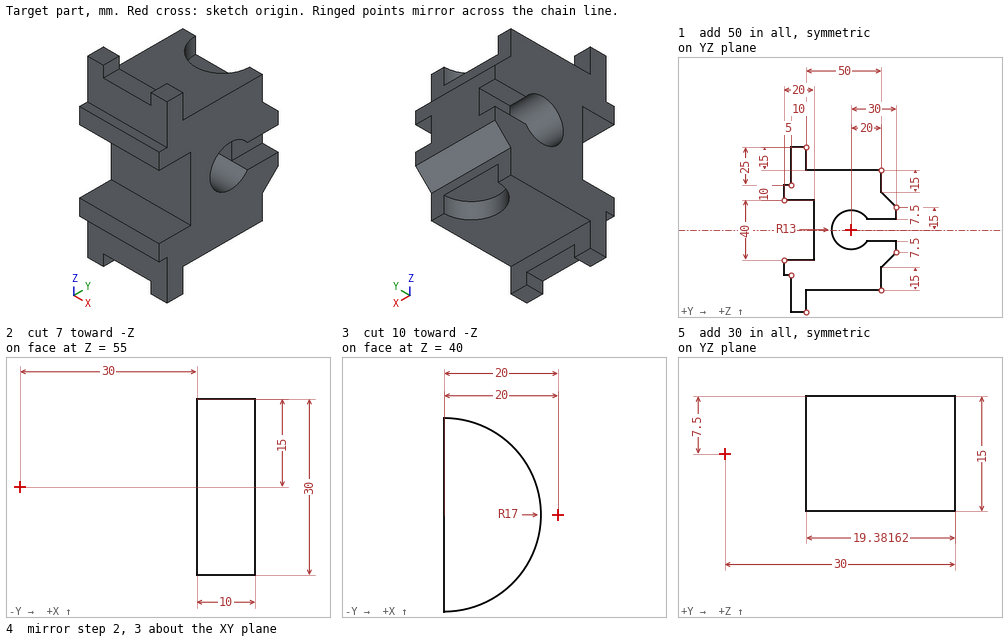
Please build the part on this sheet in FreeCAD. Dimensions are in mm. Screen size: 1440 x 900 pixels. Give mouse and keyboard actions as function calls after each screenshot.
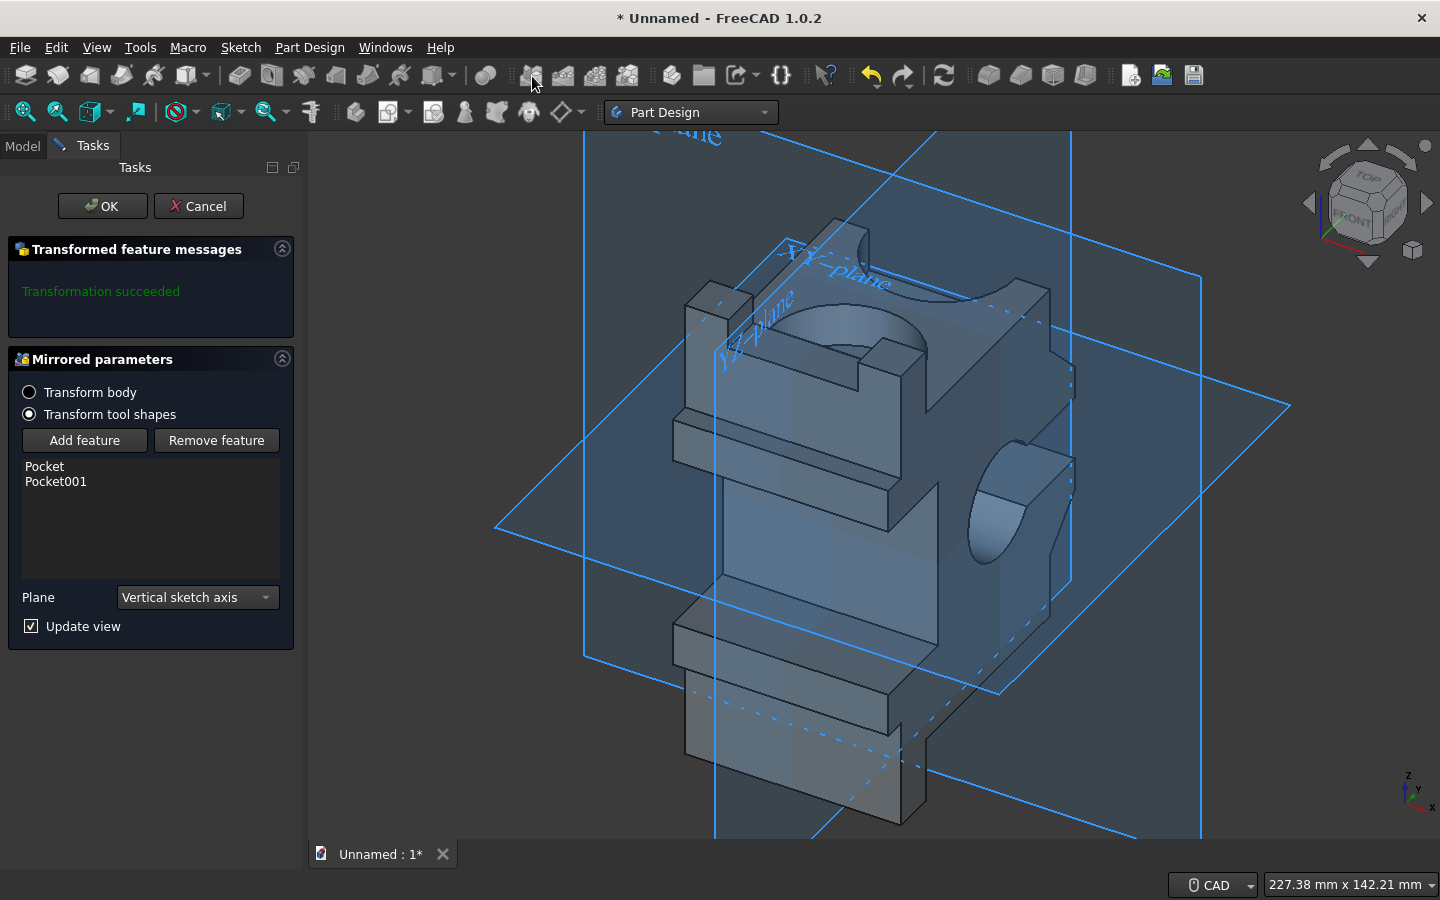
click(198, 598)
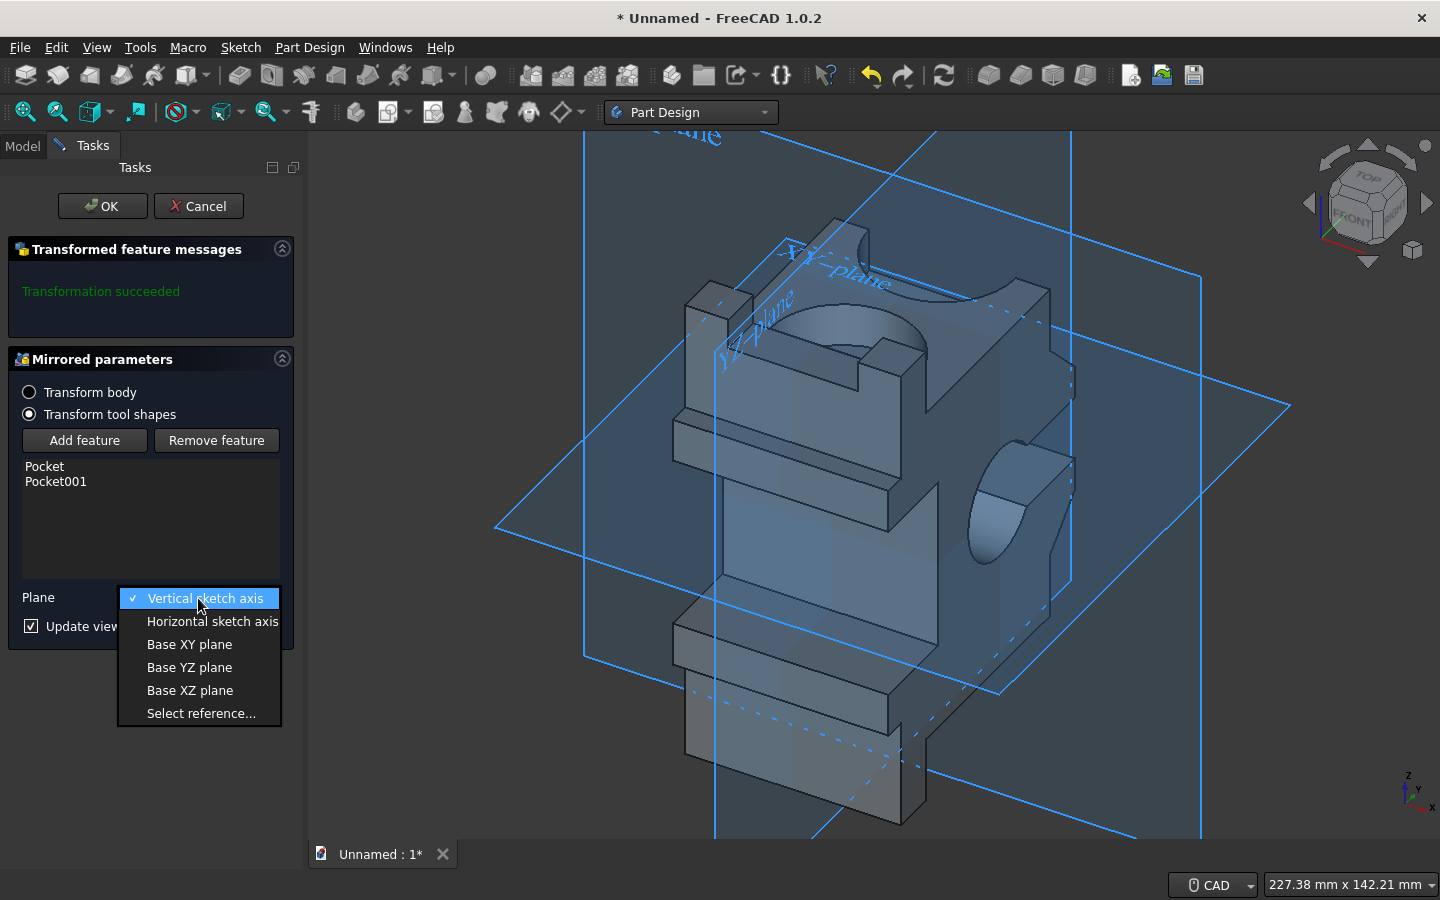
click(198, 644)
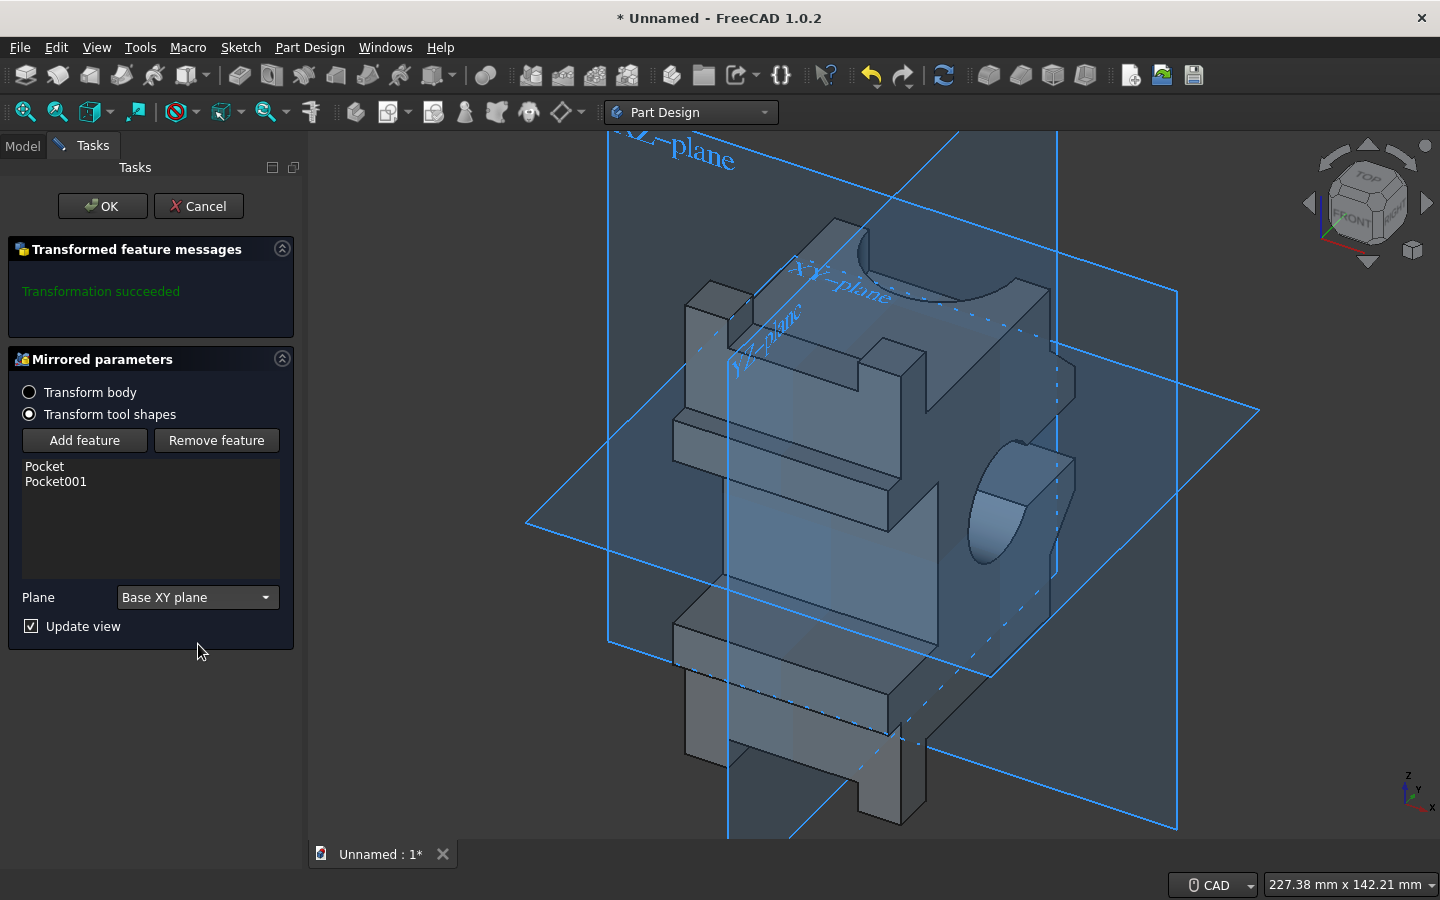
click(103, 206)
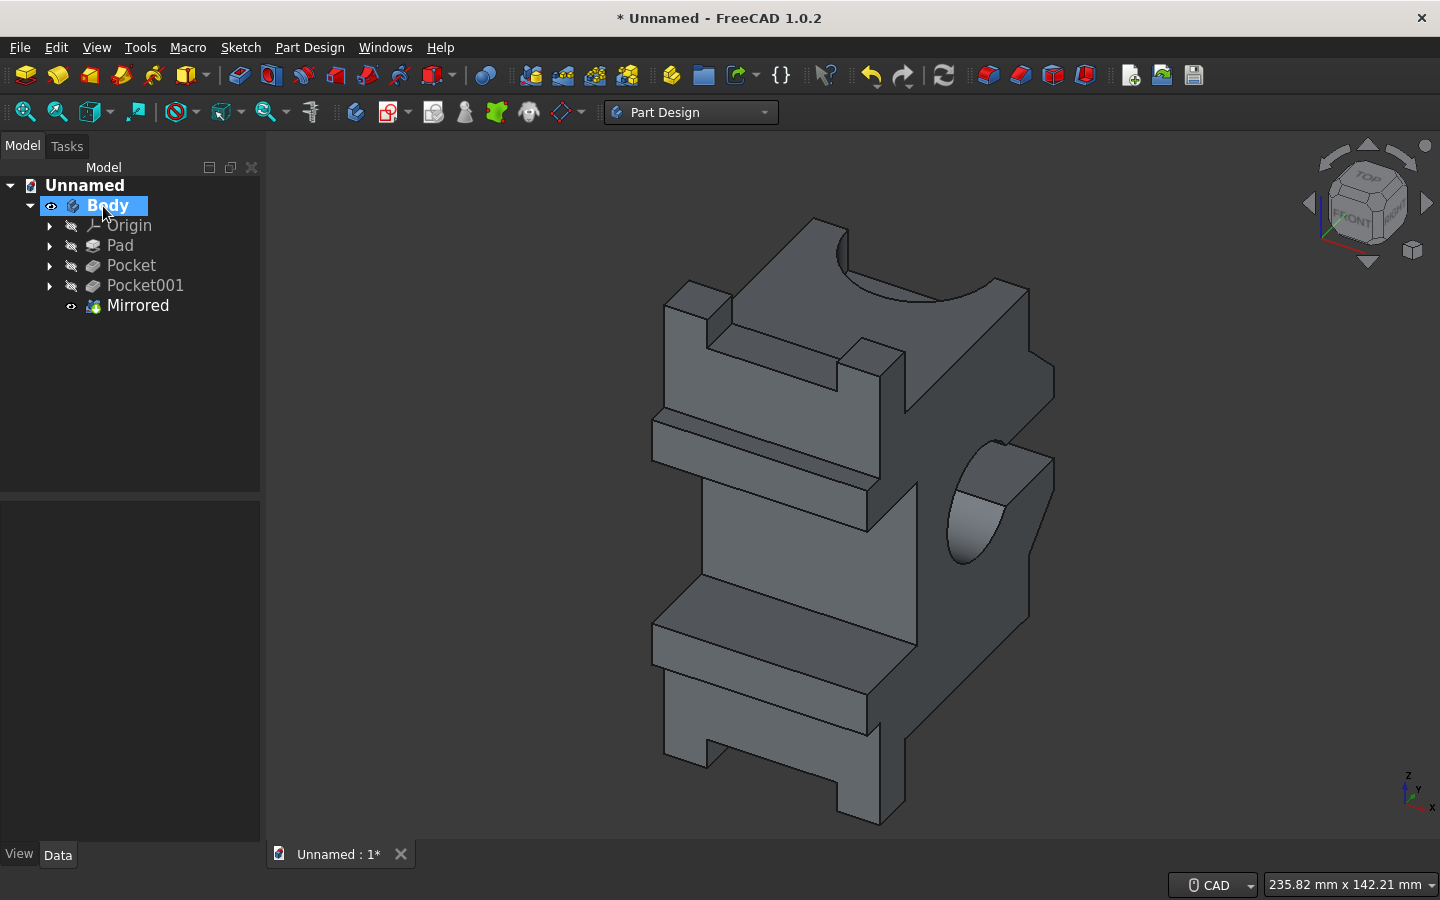
click(388, 112)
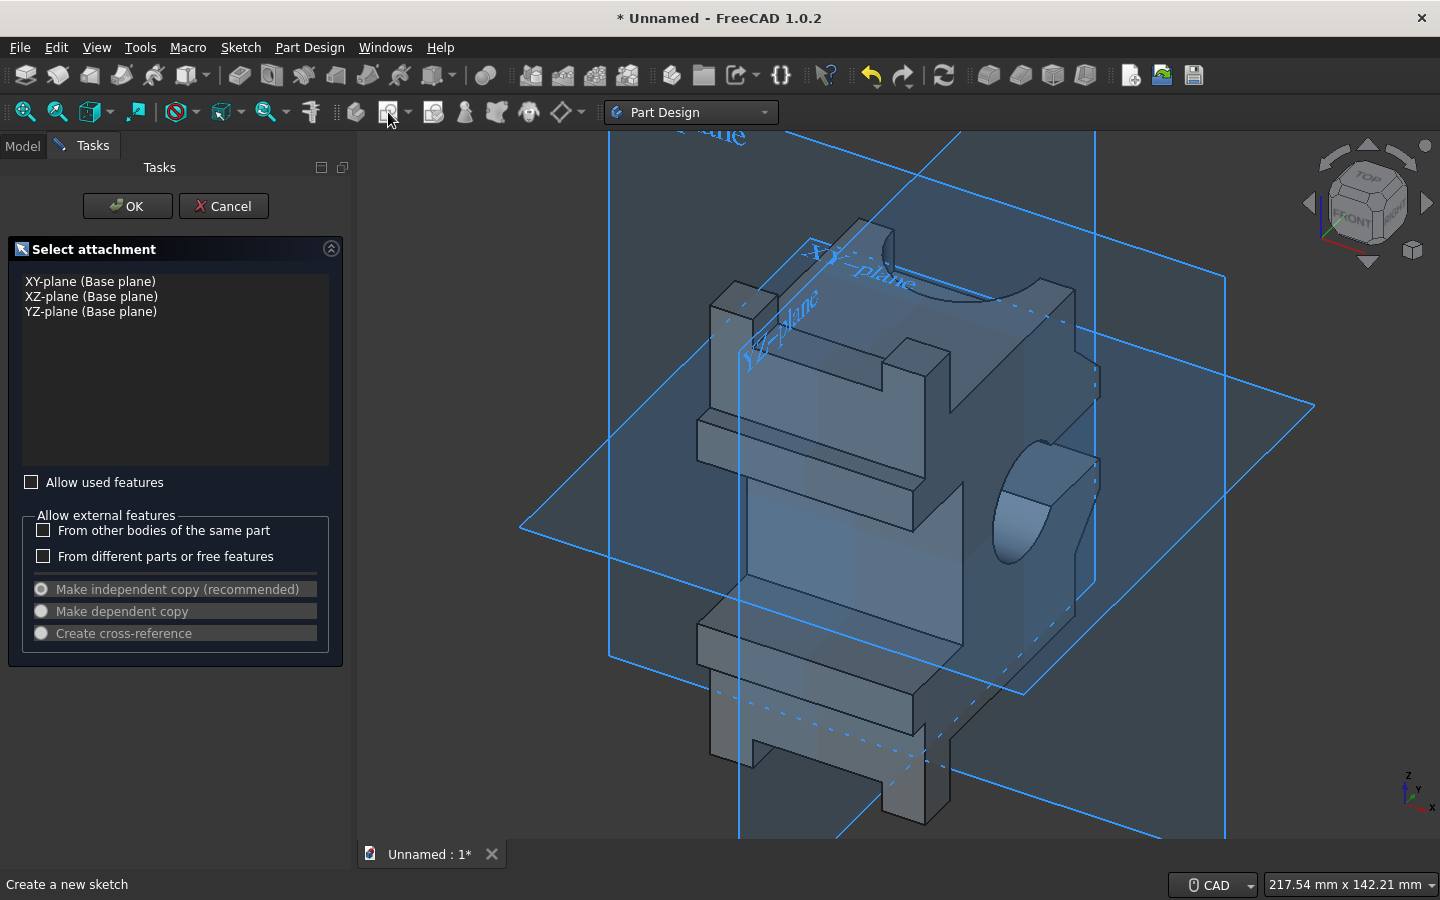
click(82, 312)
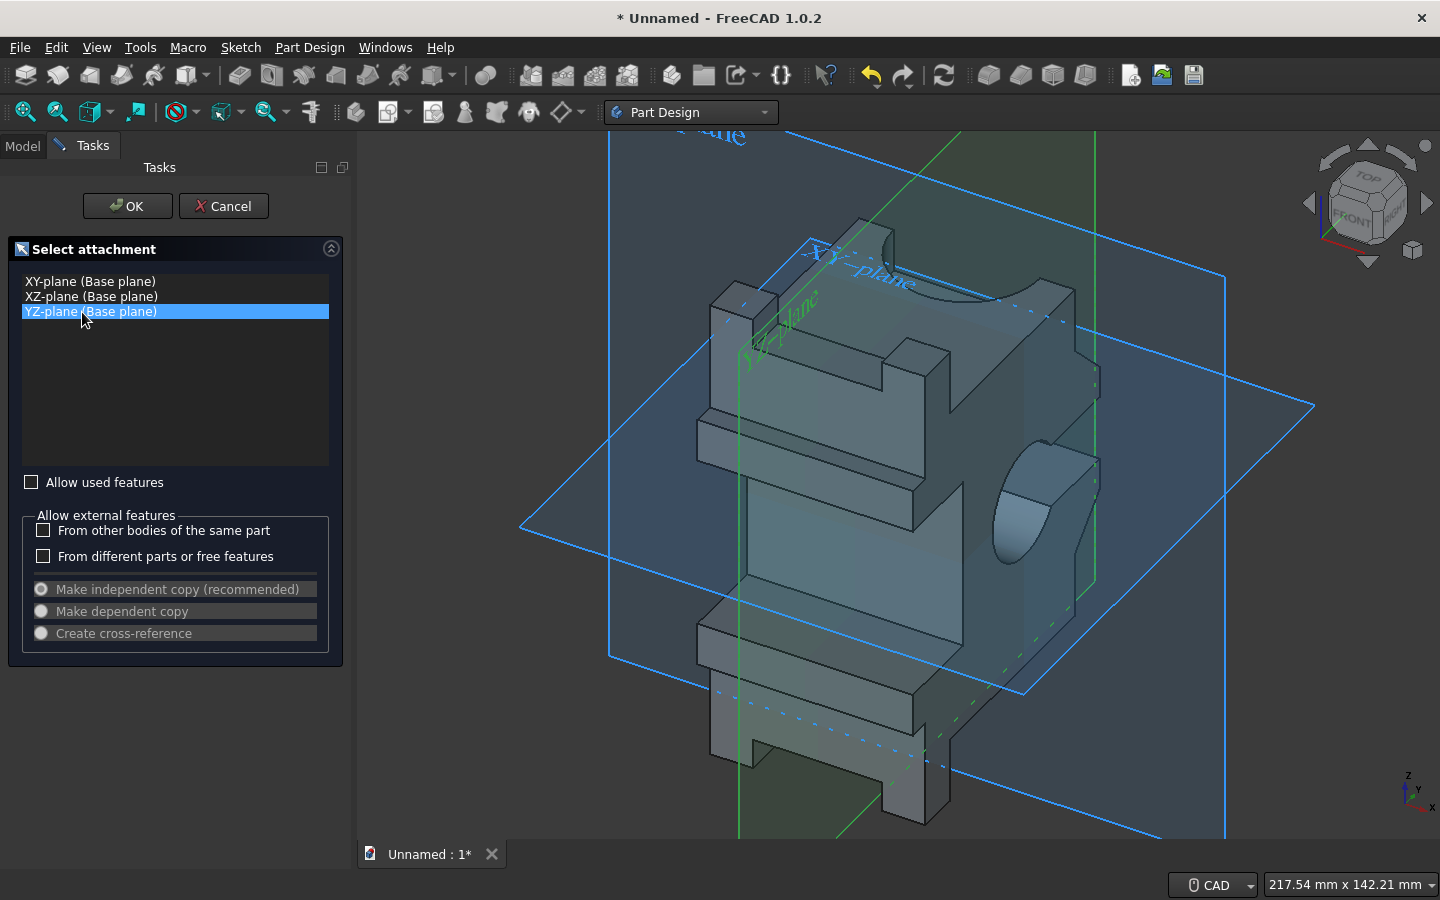
click(128, 206)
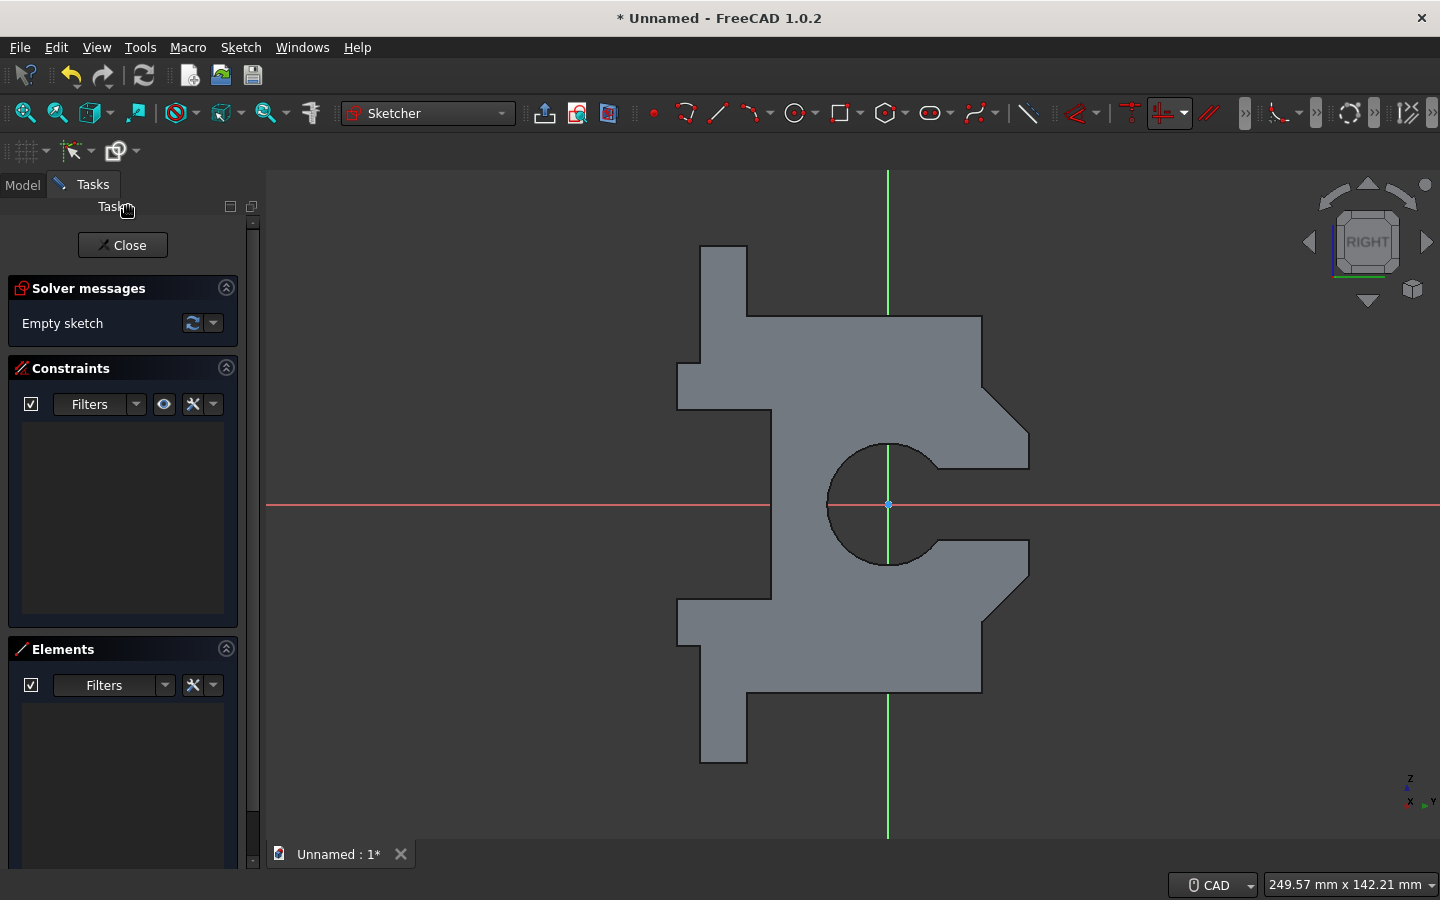
click(610, 114)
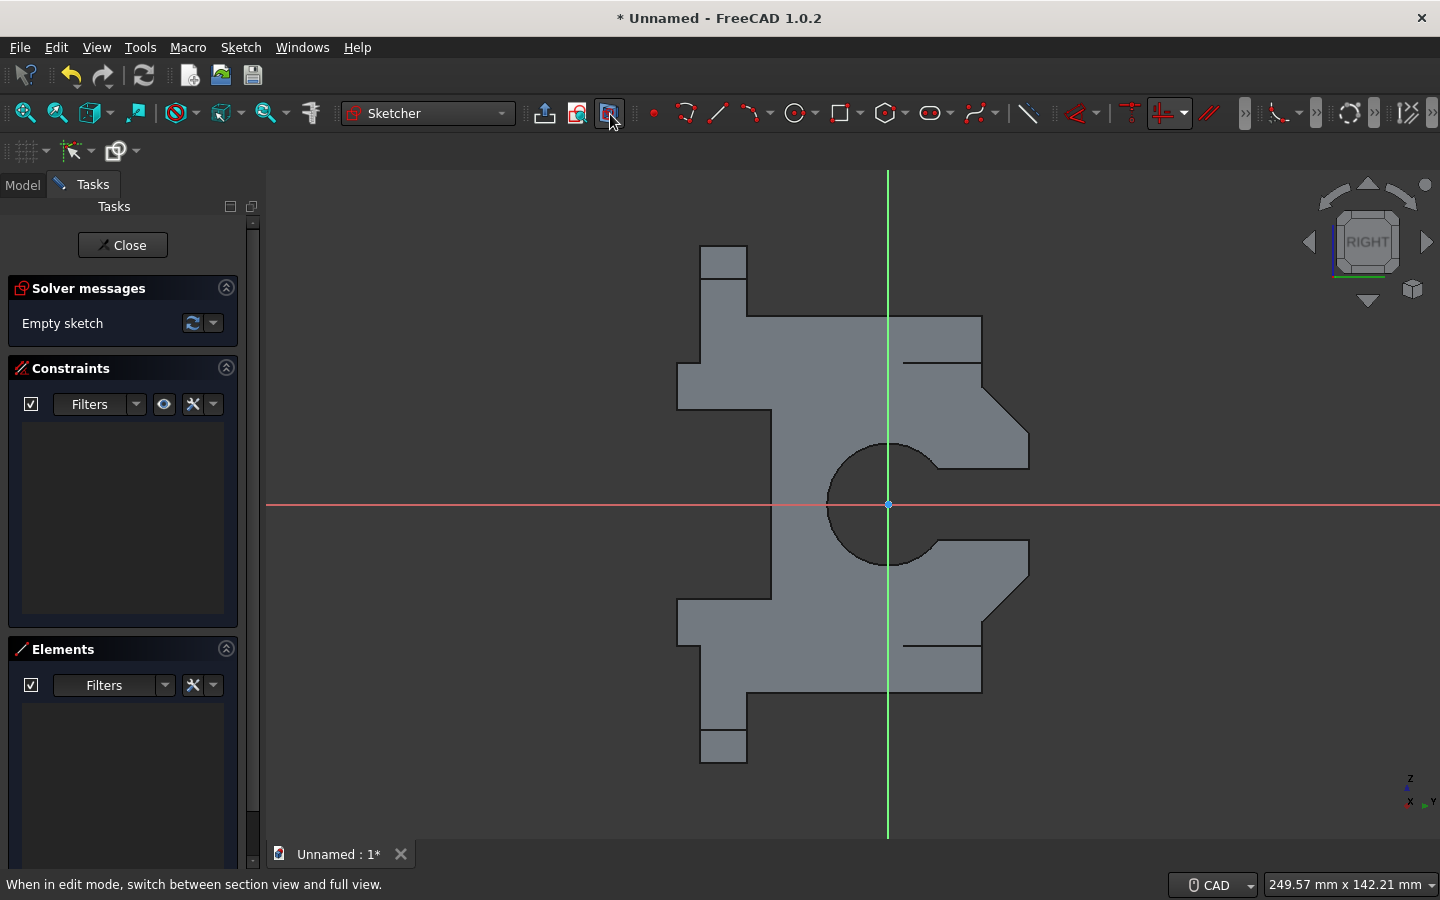
scroll(1003, 505, up, 8)